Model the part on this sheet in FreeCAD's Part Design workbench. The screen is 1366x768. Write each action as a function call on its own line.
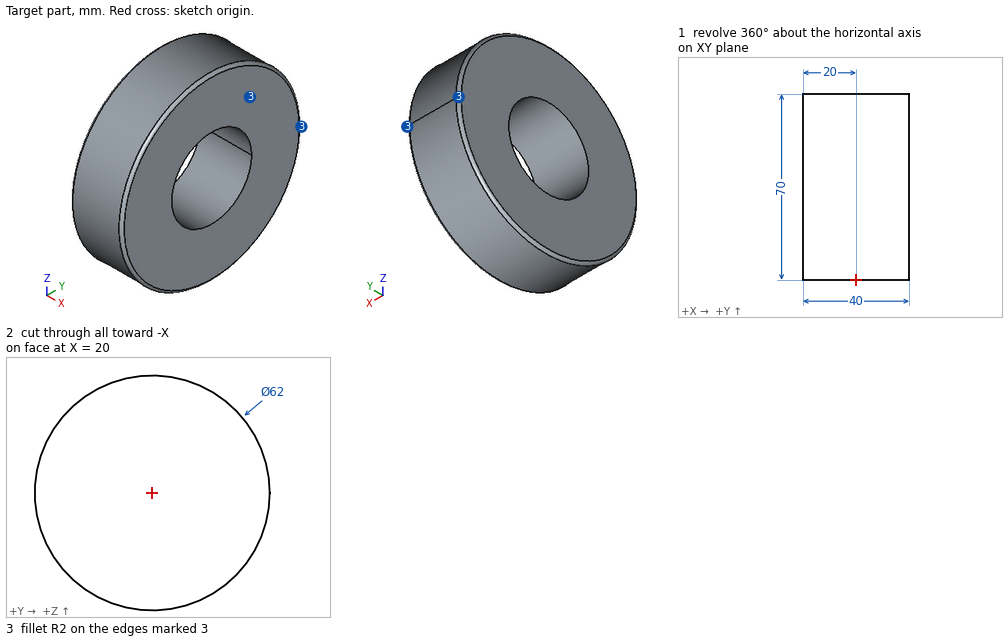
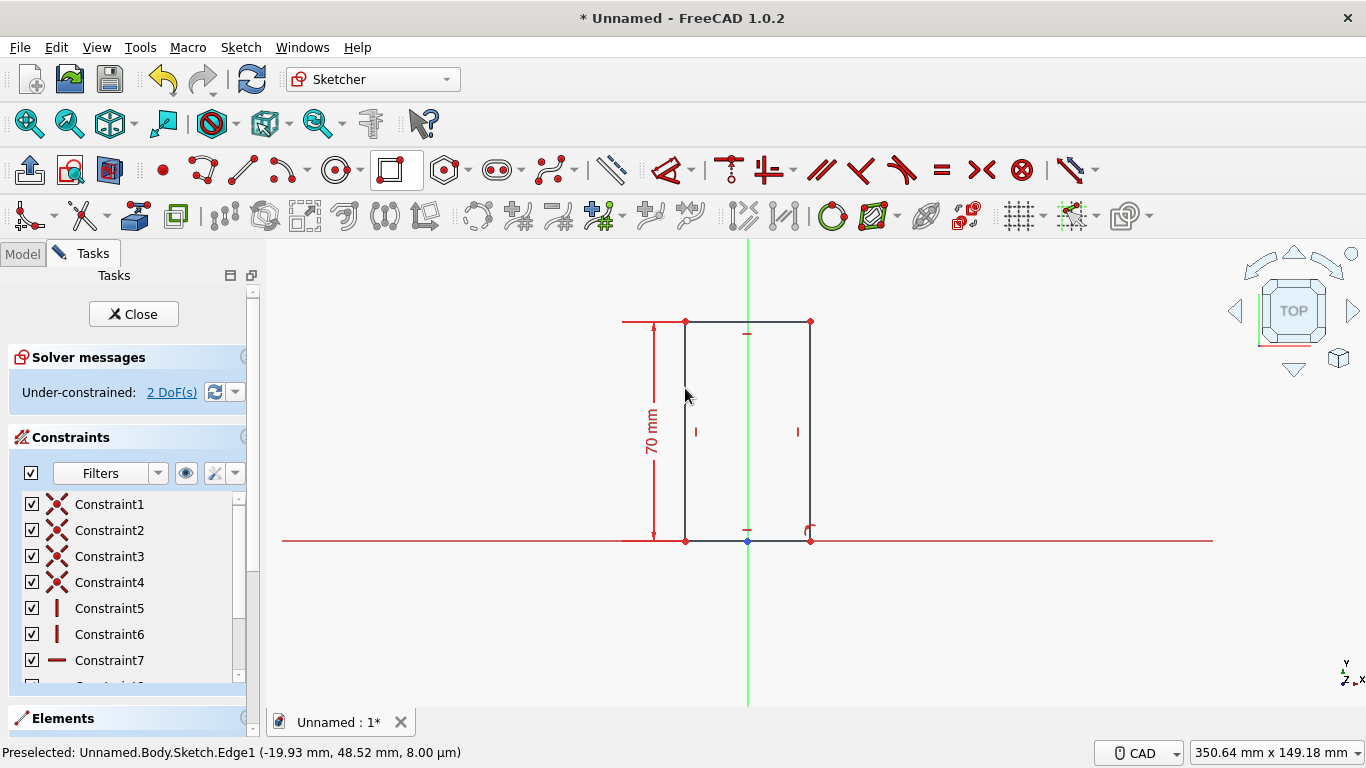
click(722, 541)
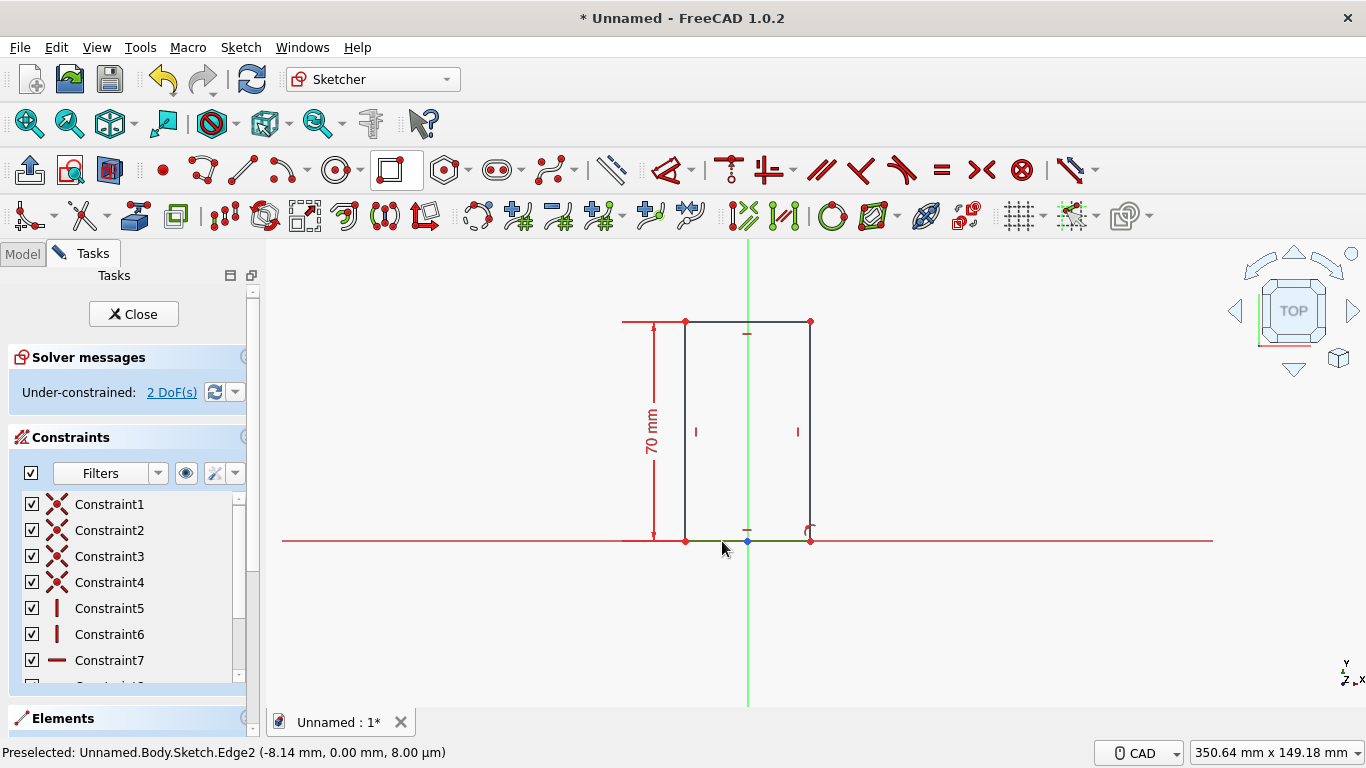
key(l)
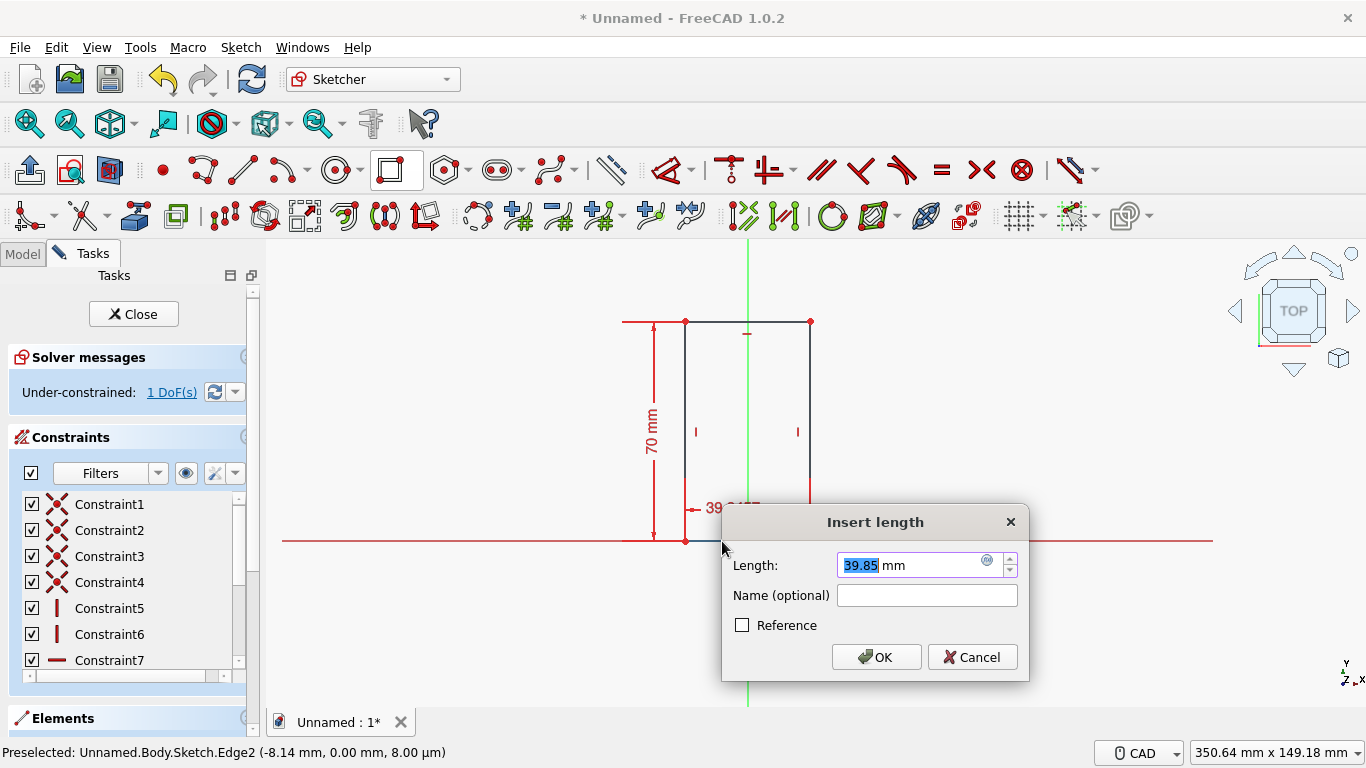
text(40)
key(Return)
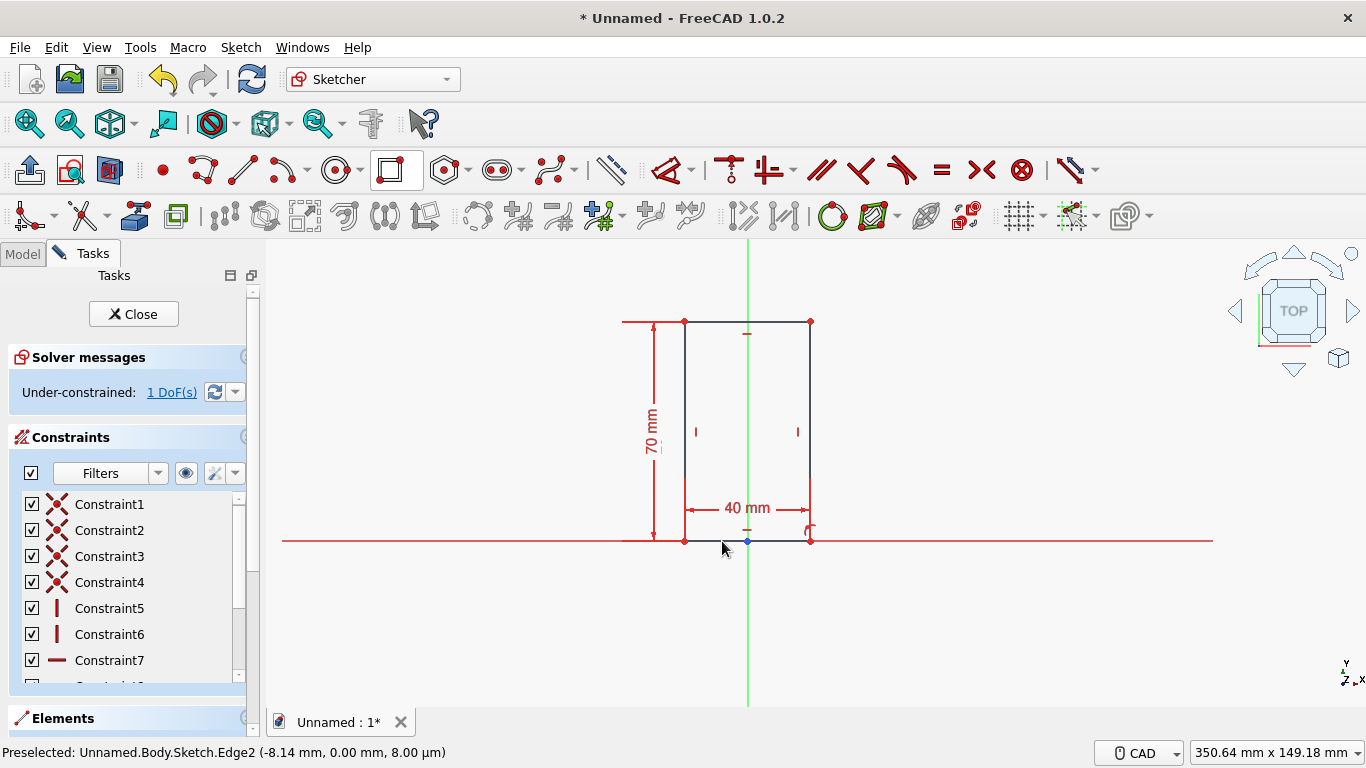
click(685, 322)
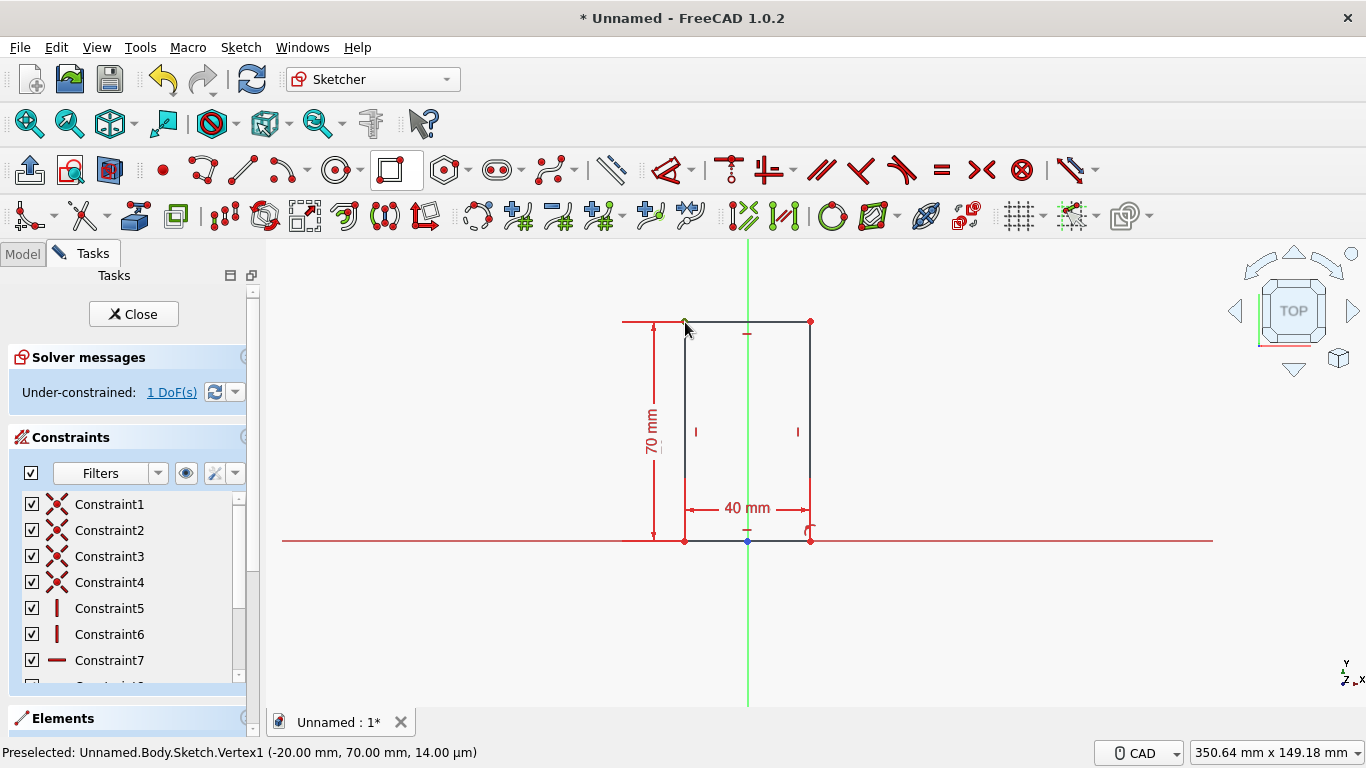
key(l)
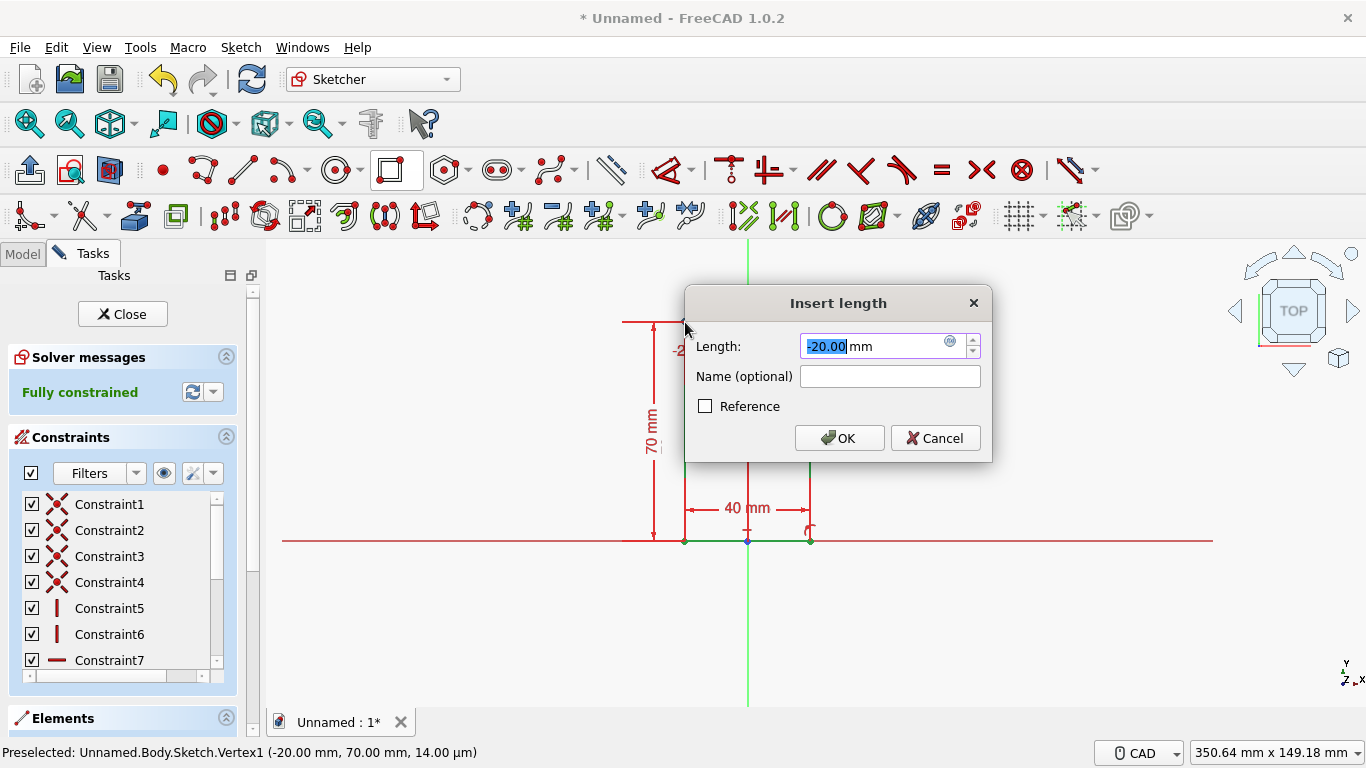
text(-20)
key(Return)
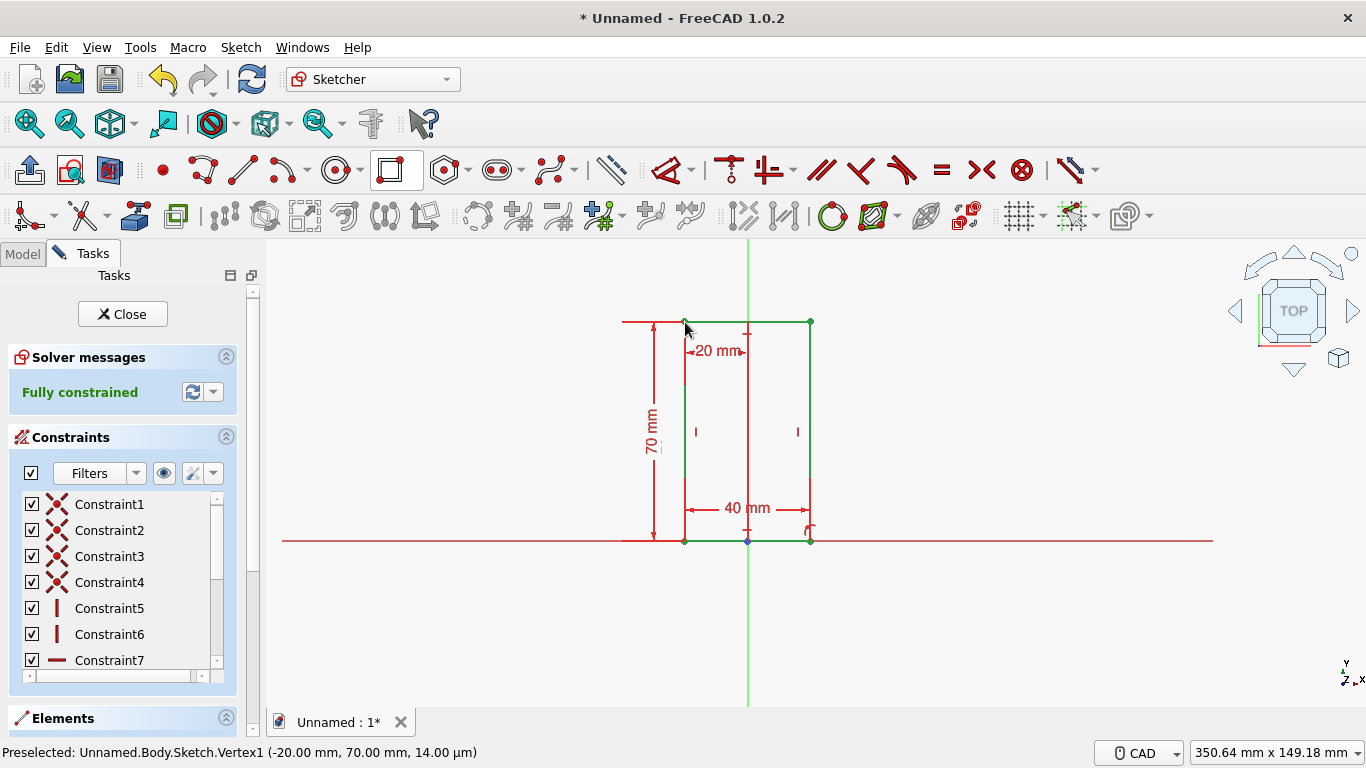
click(123, 314)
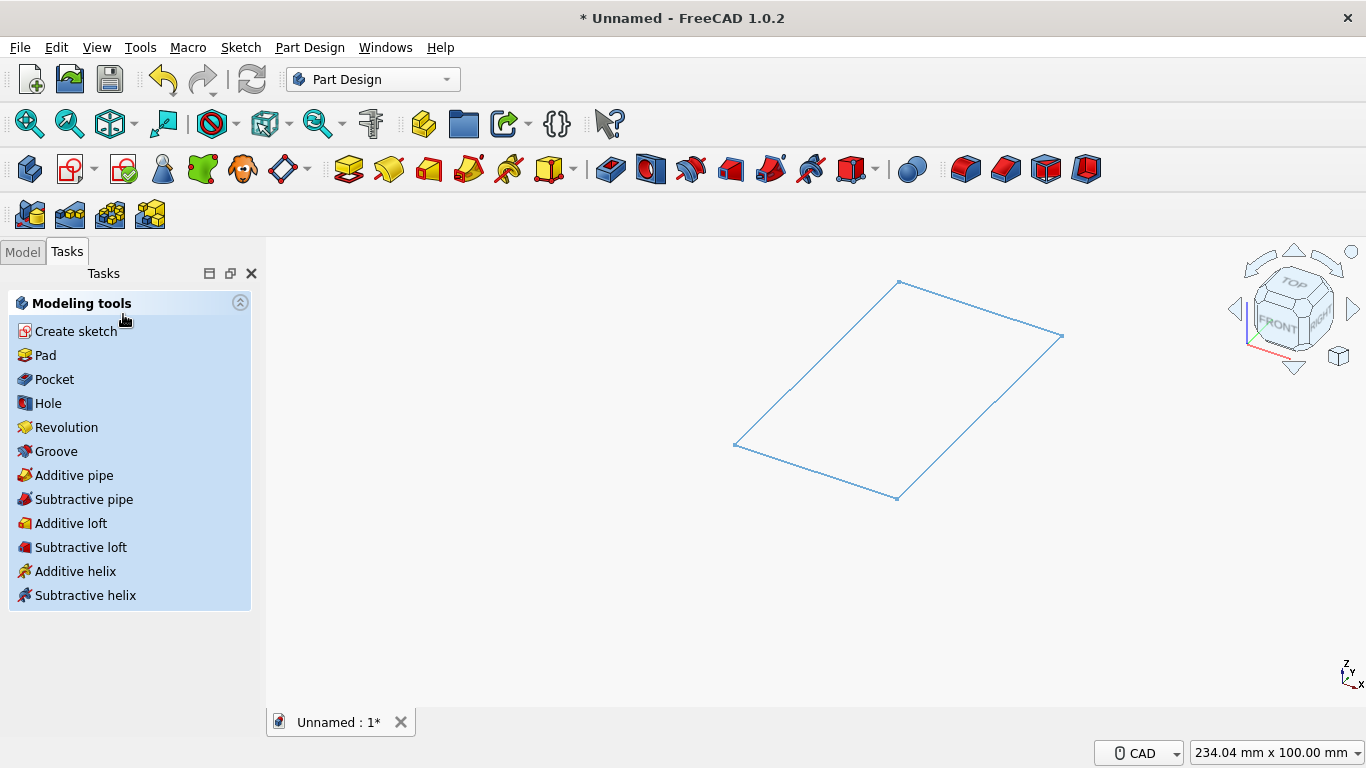
click(390, 170)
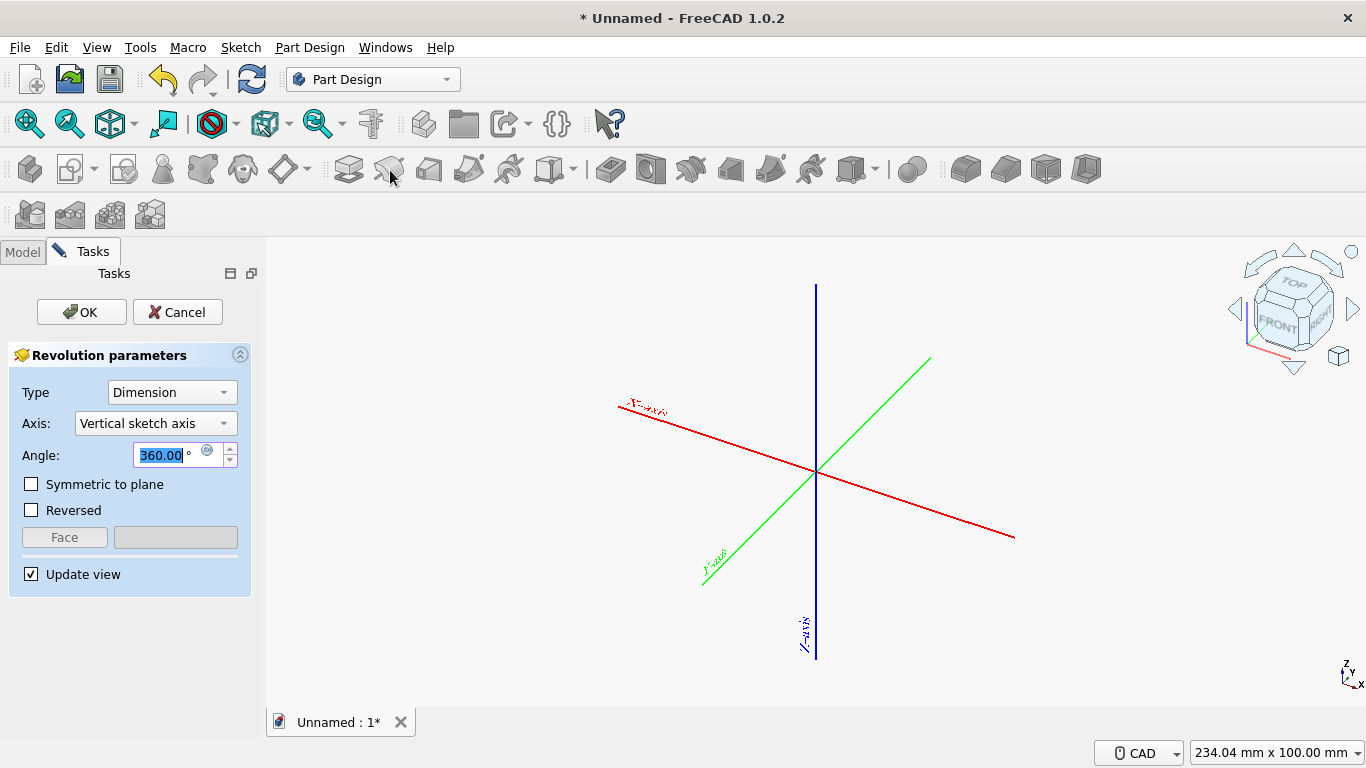
click(156, 424)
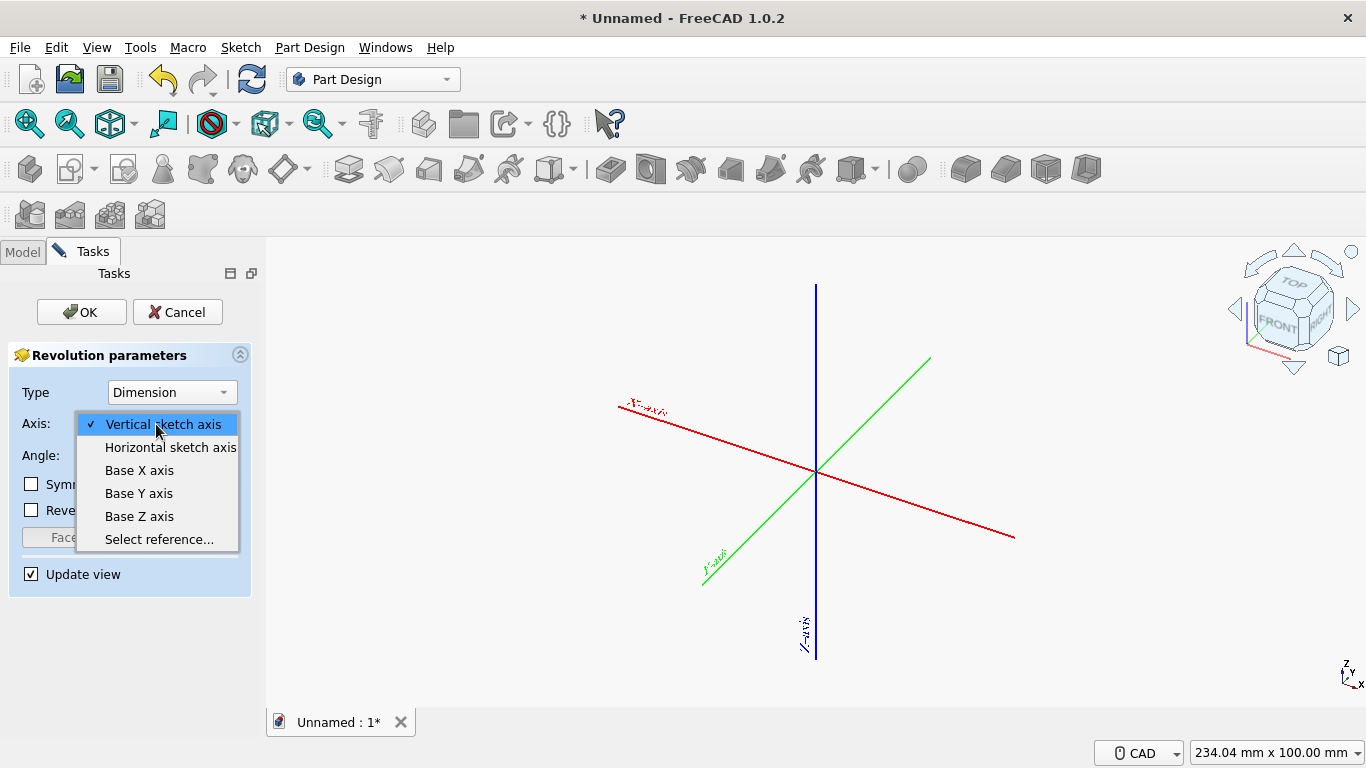
click(156, 448)